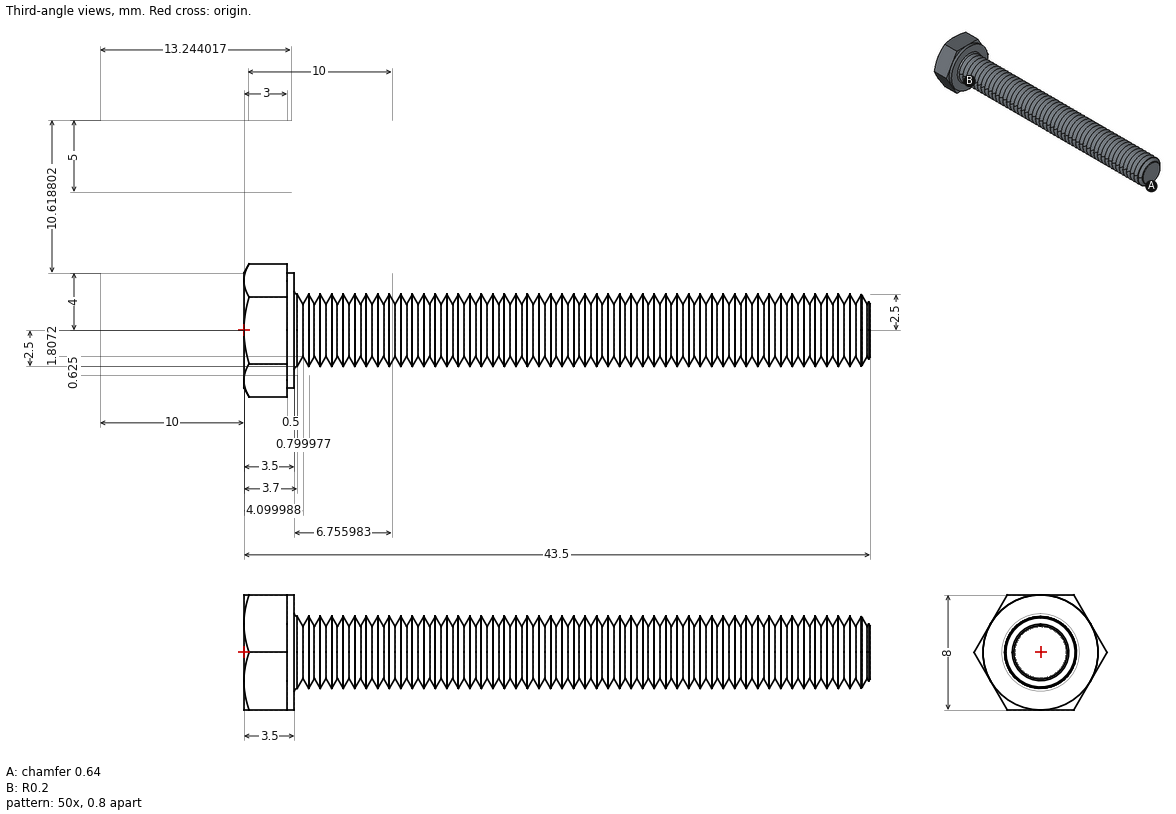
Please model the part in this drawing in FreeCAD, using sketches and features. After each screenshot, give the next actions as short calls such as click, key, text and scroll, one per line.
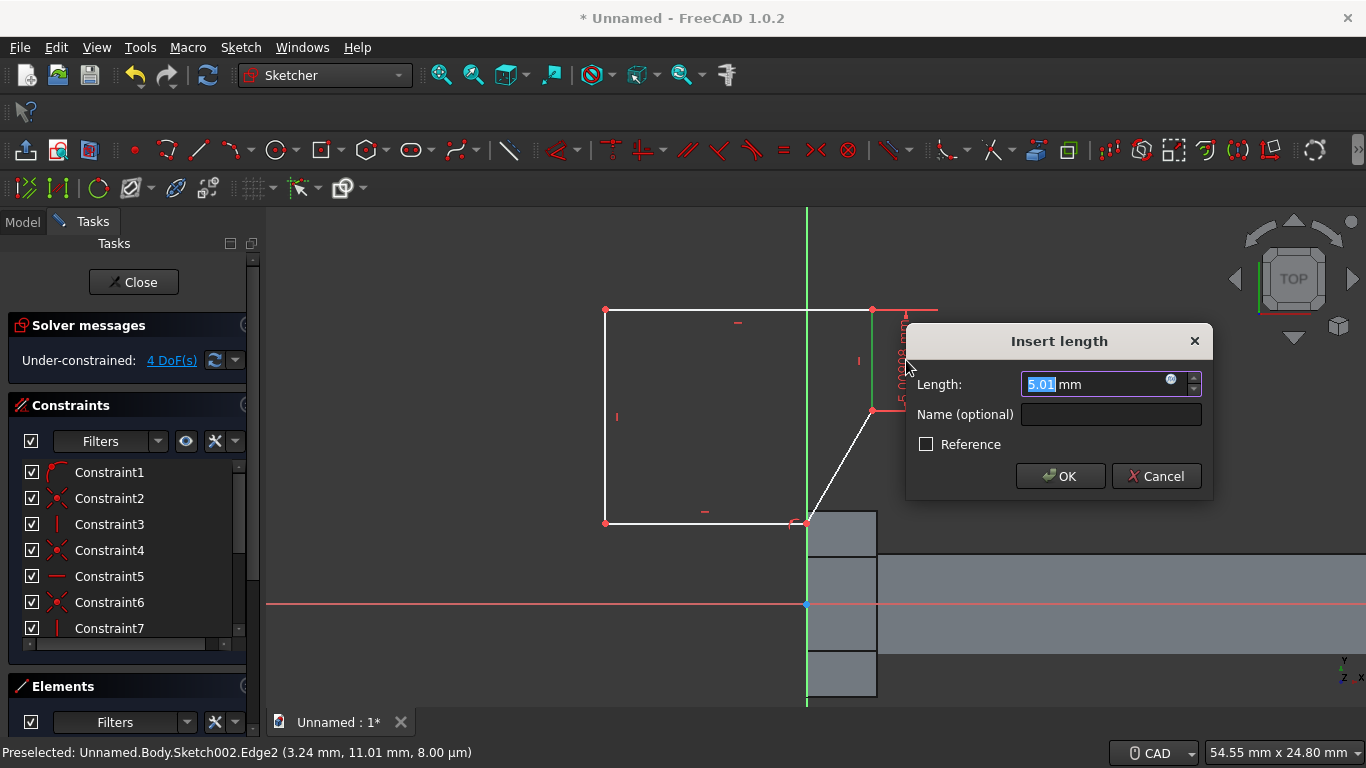
text(5)
key(Return)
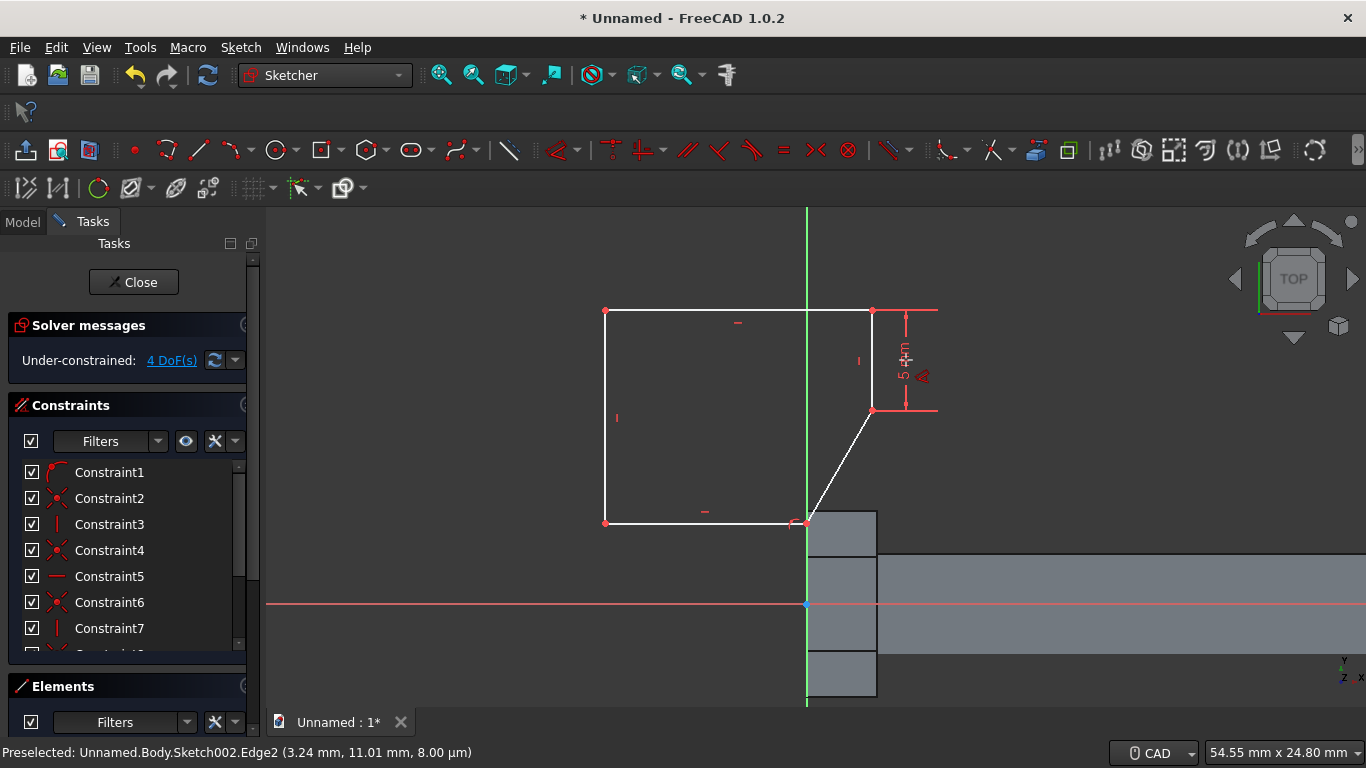
click(665, 524)
click(706, 558)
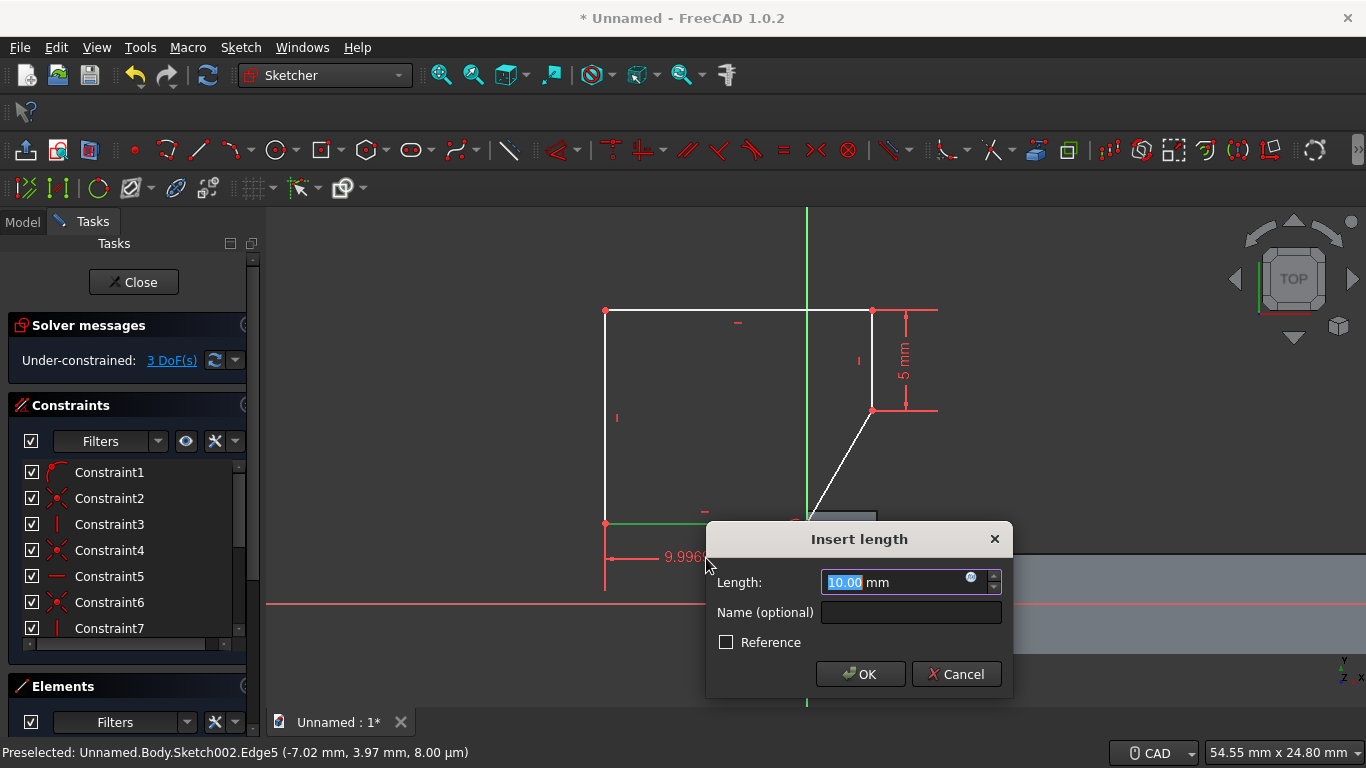
text(10)
key(Return)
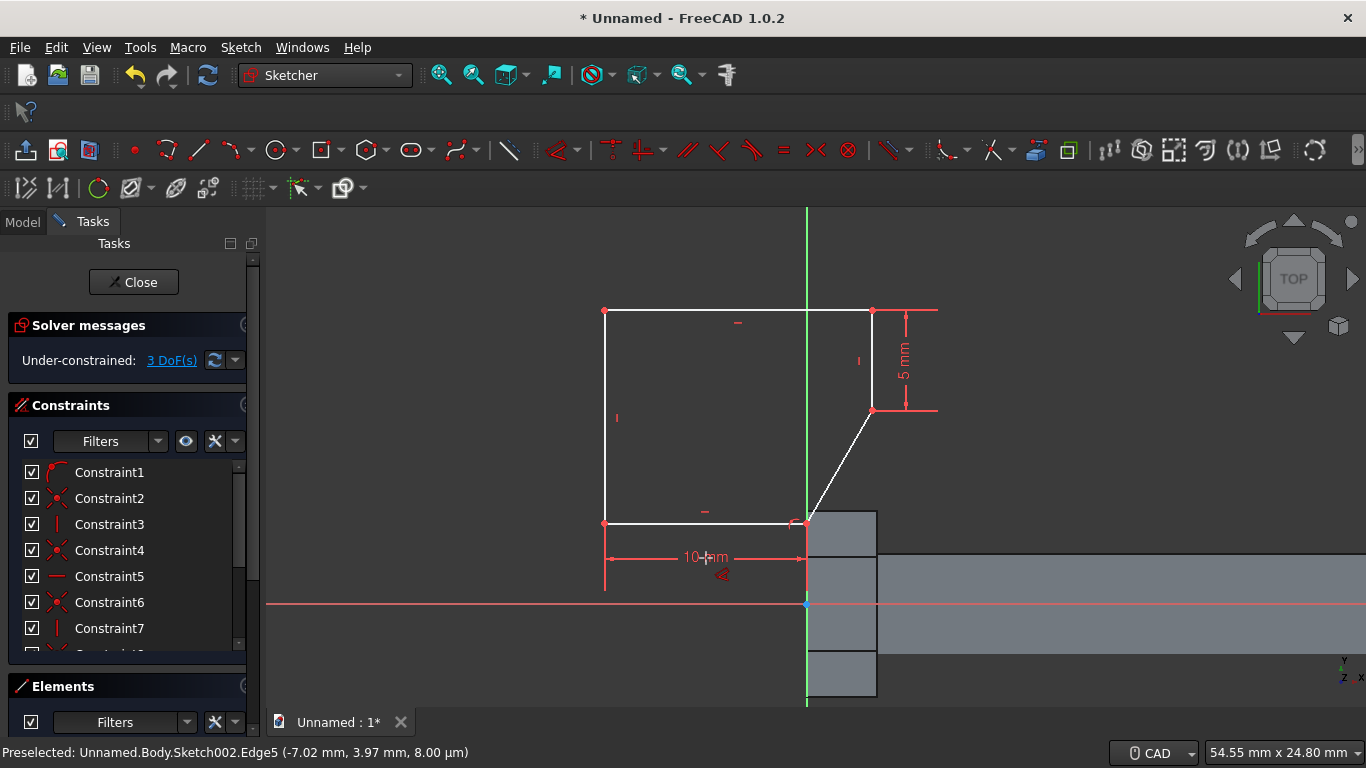
click(807, 524)
click(841, 564)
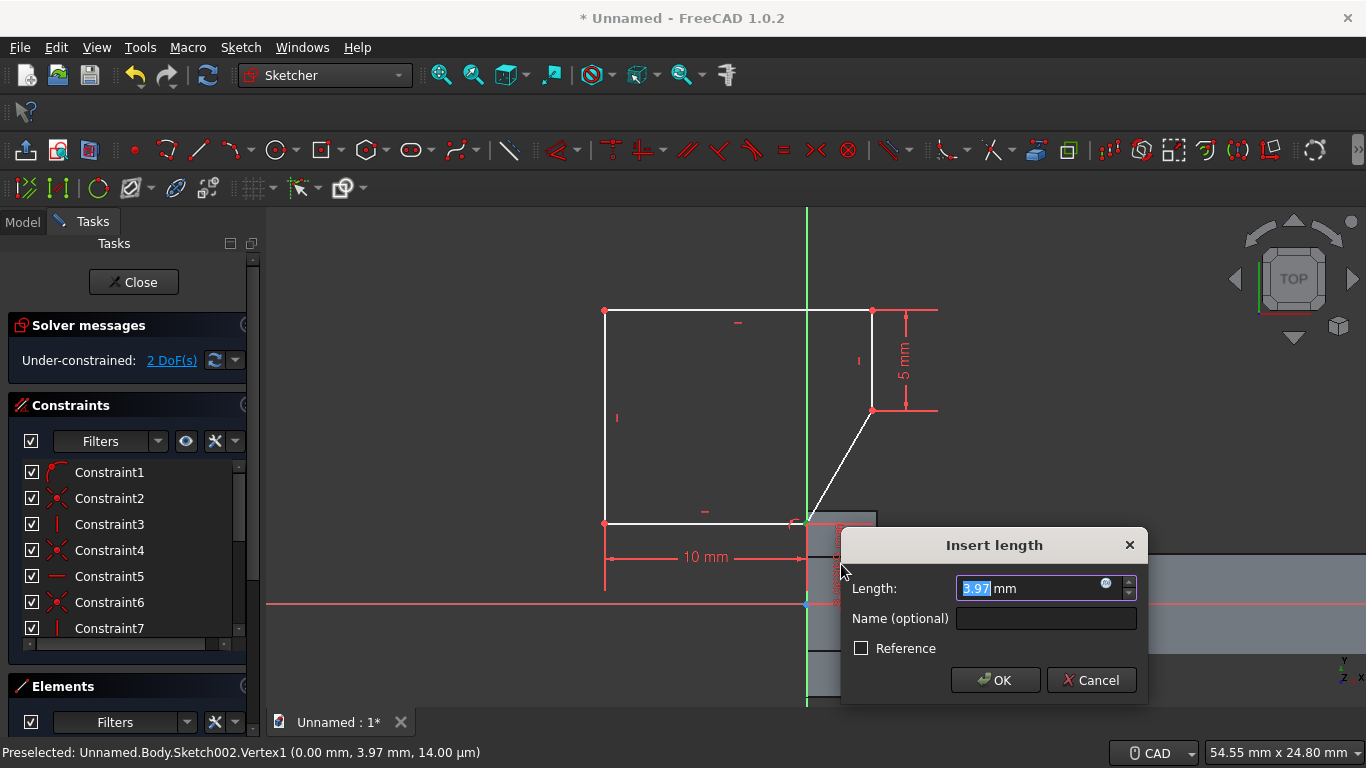
text(4)
key(Return)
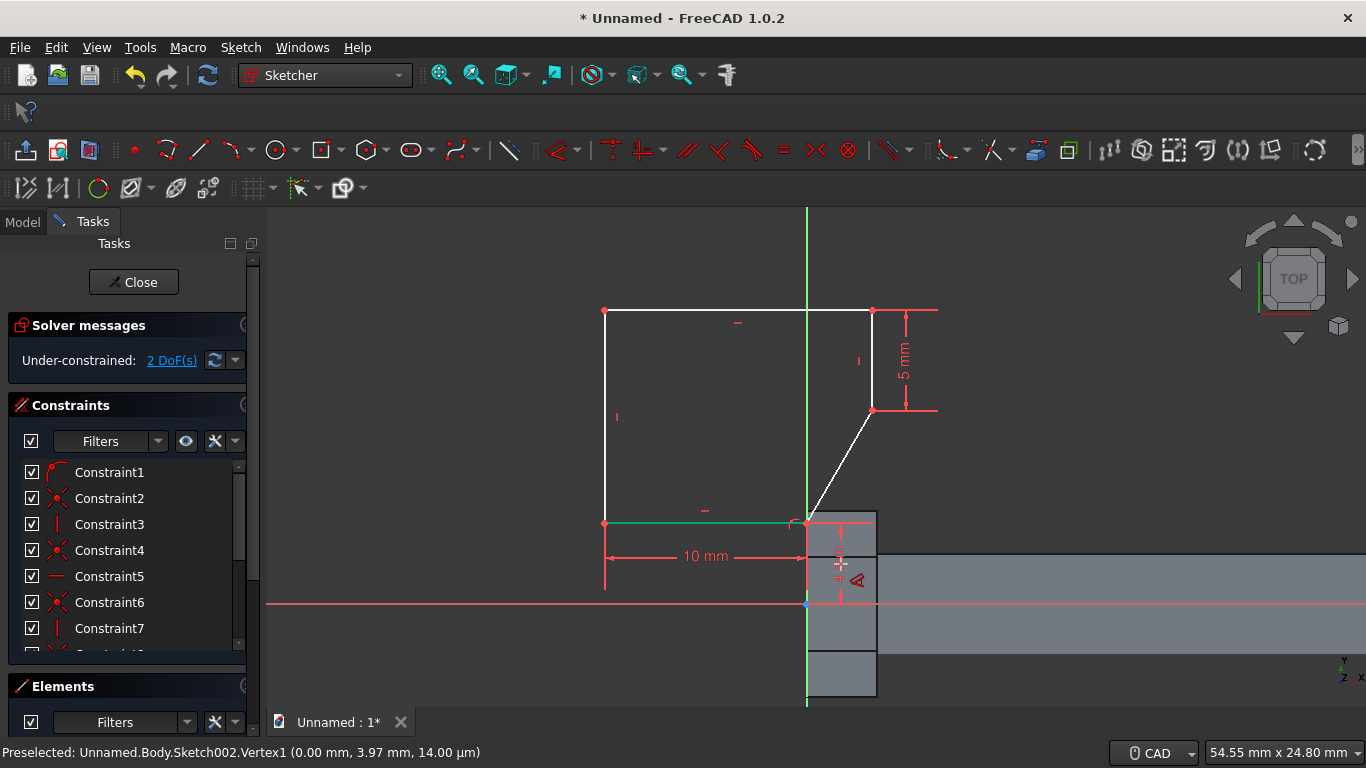
click(792, 310)
click(738, 276)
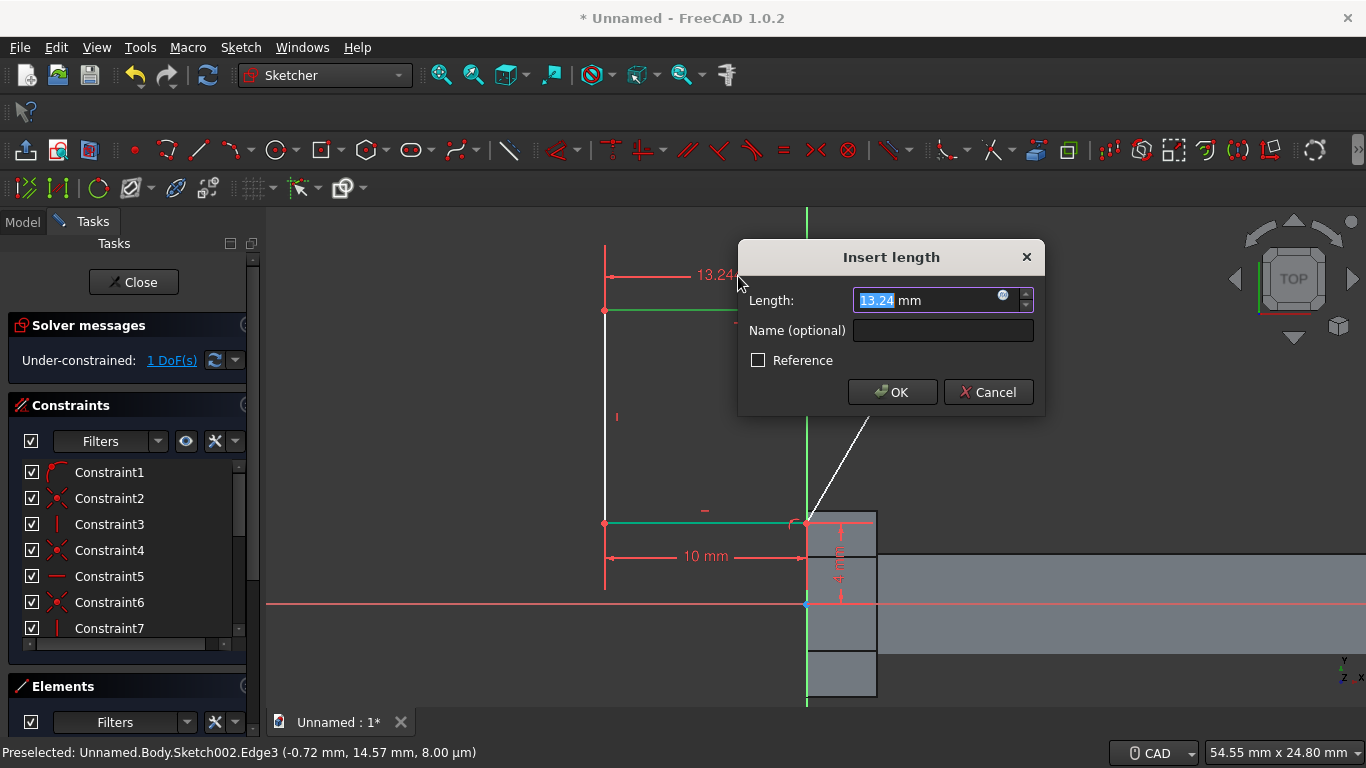
text(13.244017)
key(Return)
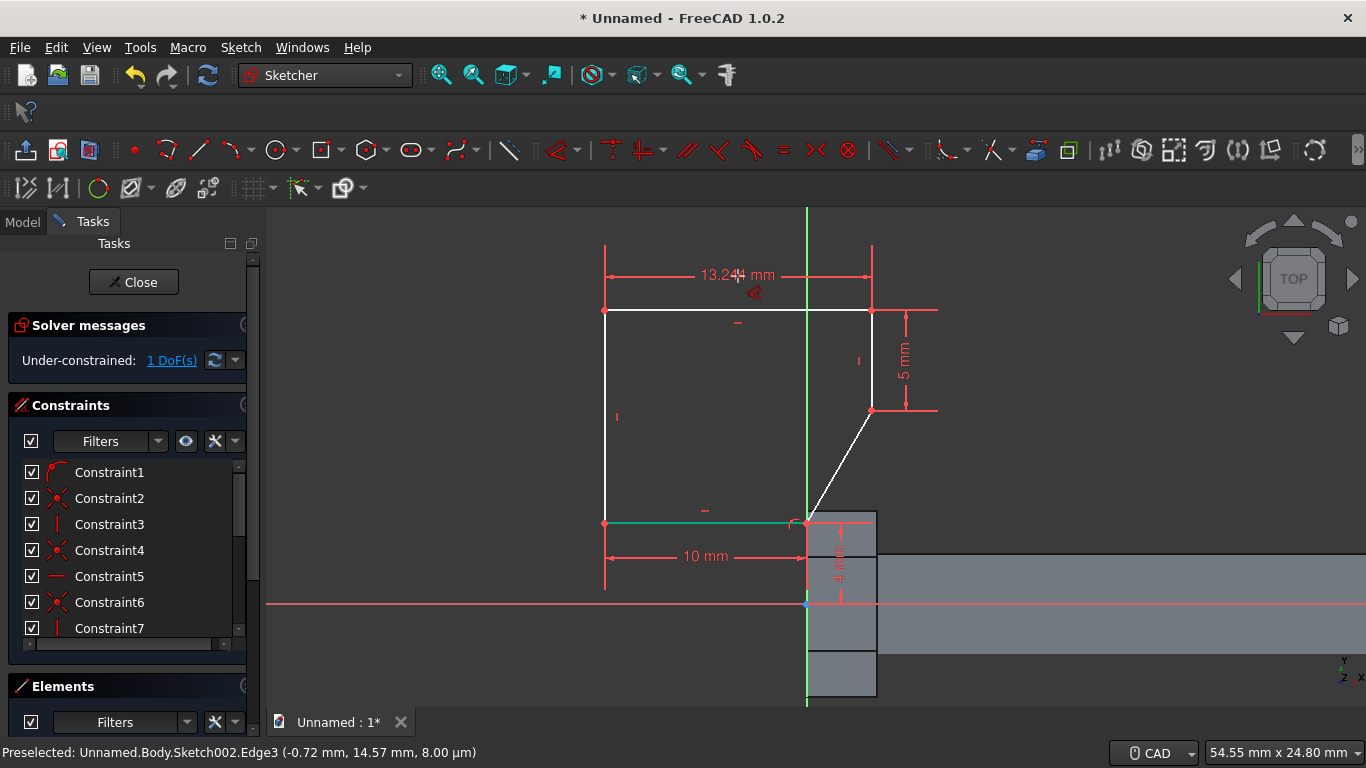
click(605, 374)
click(571, 417)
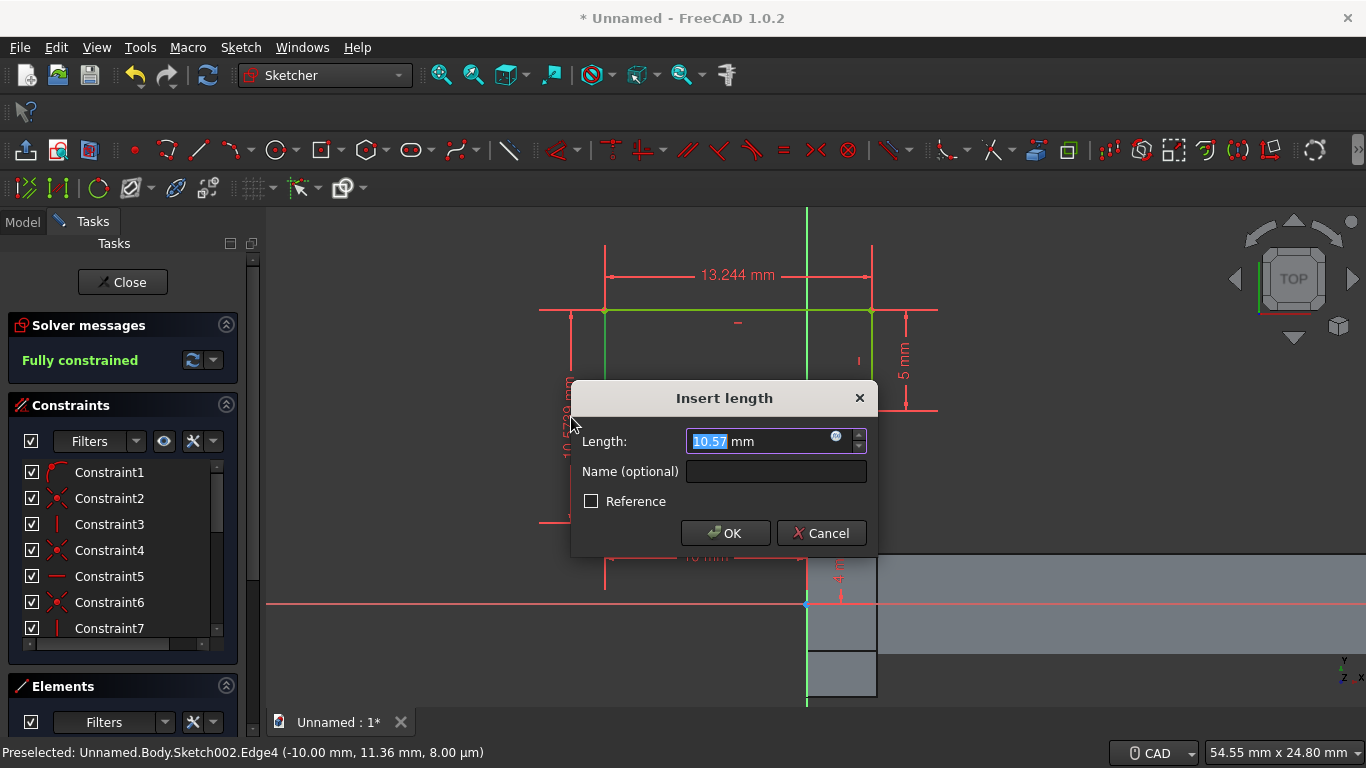
text(10.618802)
key(Return)
key(Escape)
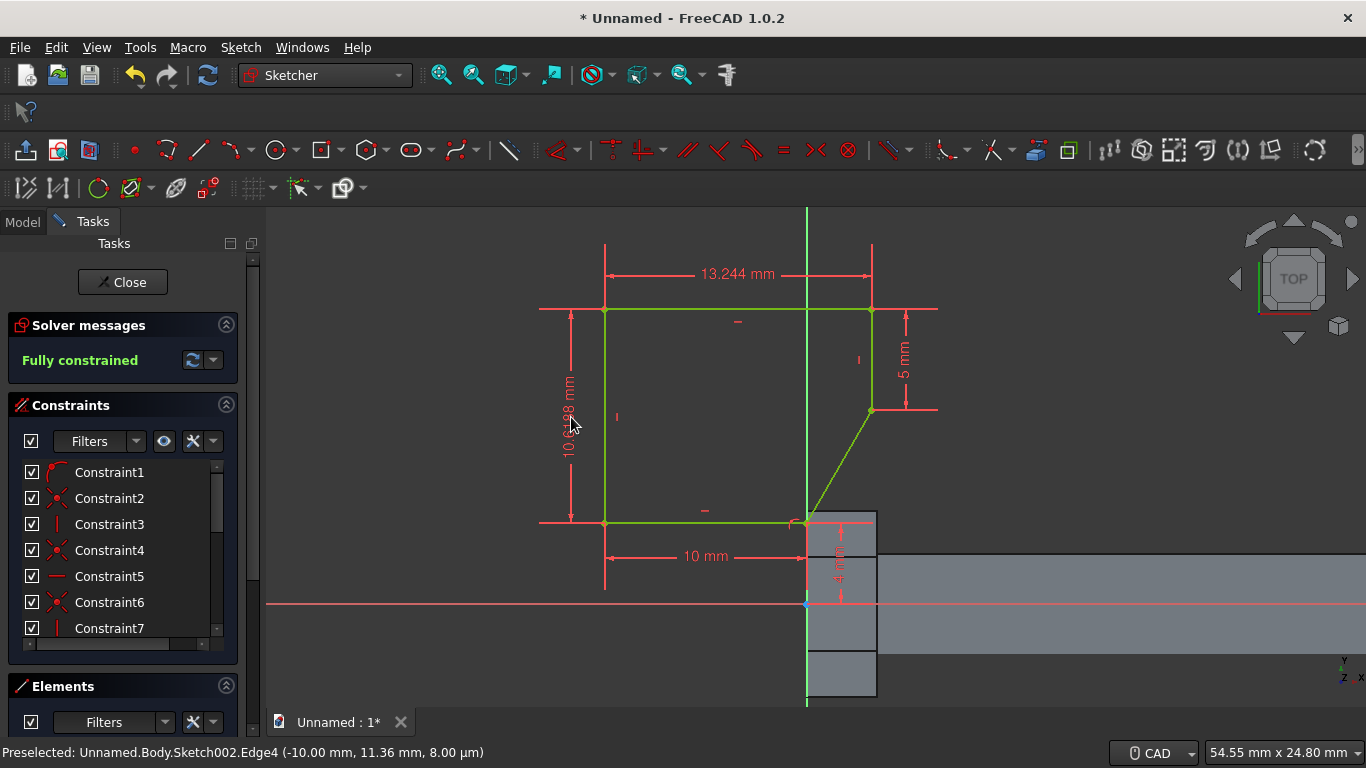
click(123, 282)